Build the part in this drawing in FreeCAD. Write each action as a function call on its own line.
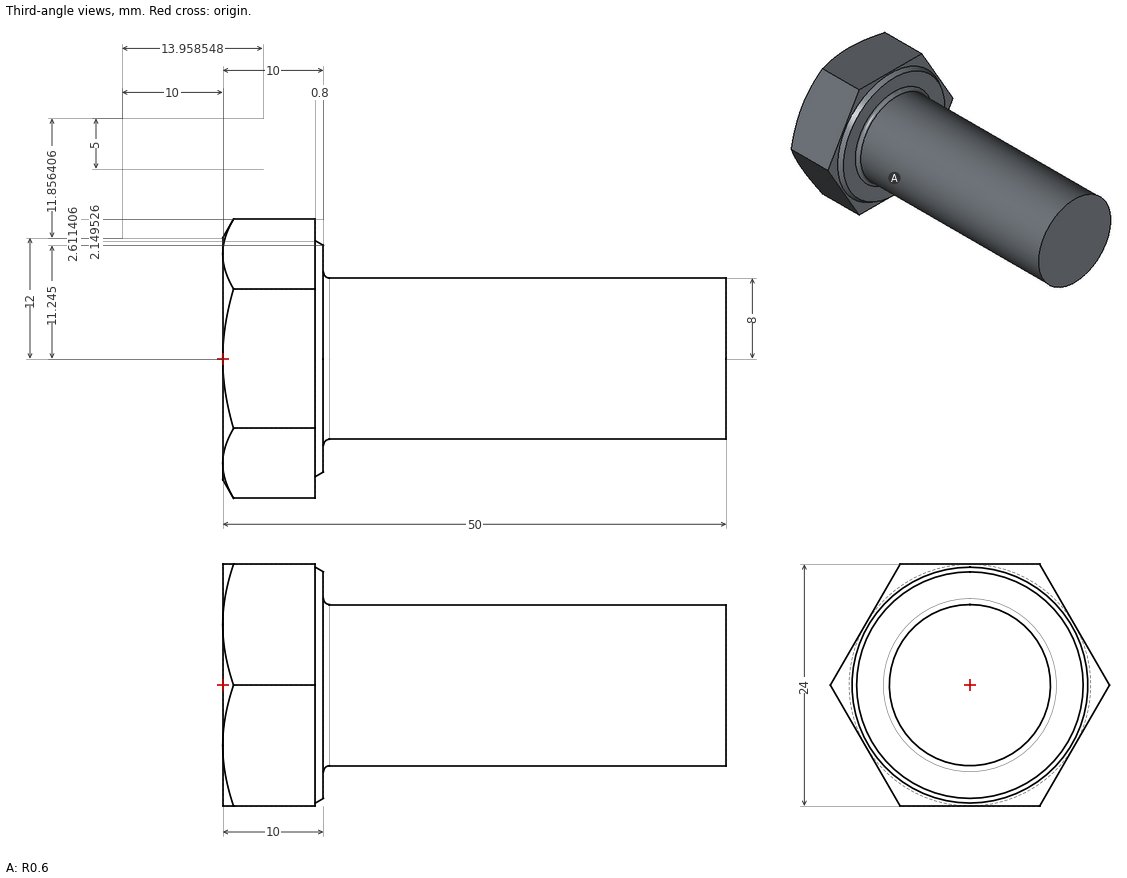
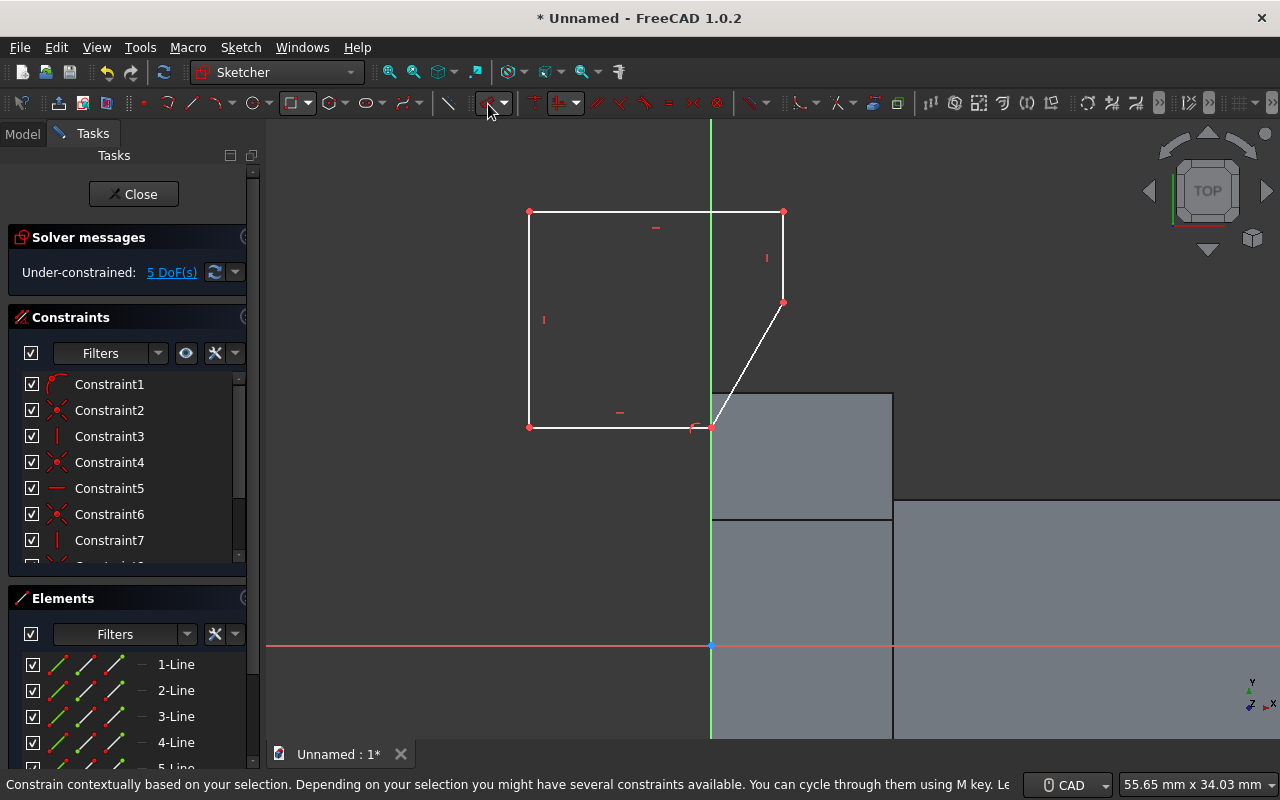
click(783, 276)
click(817, 257)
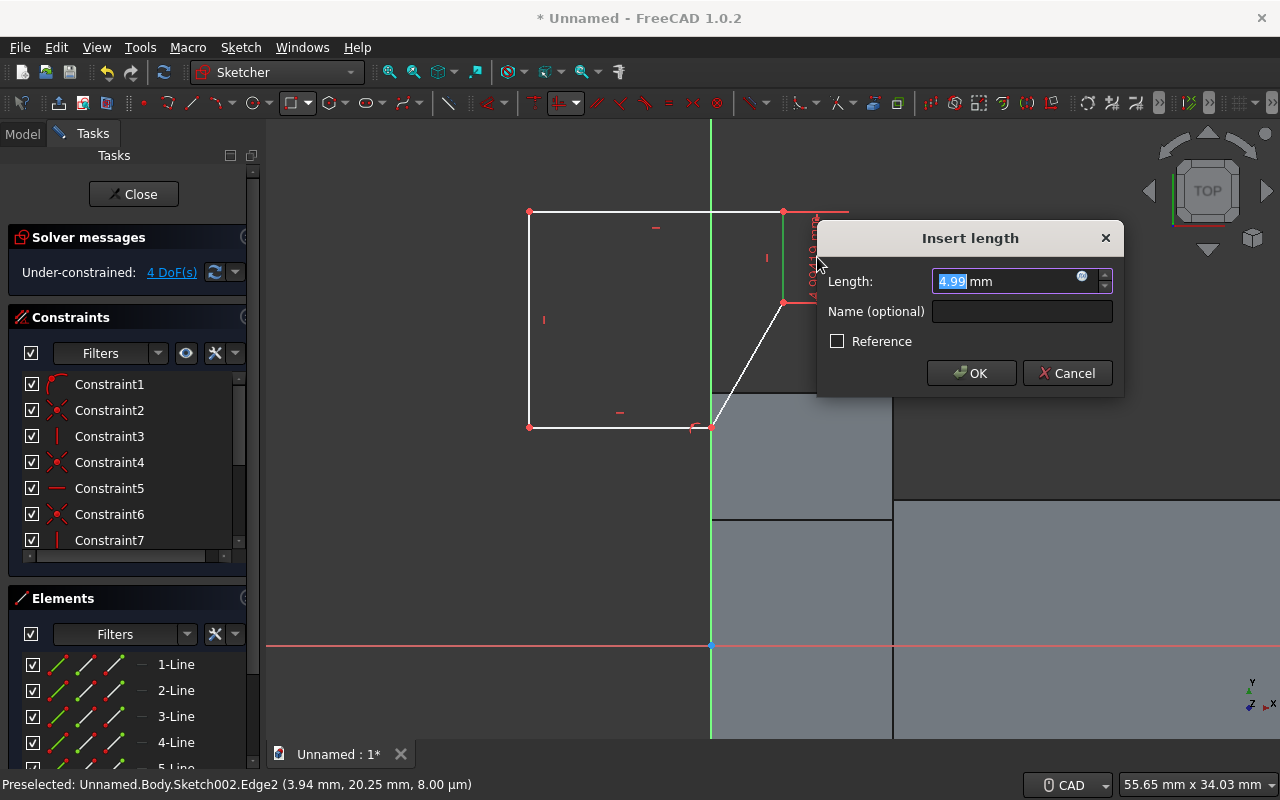
text(5)
key(Return)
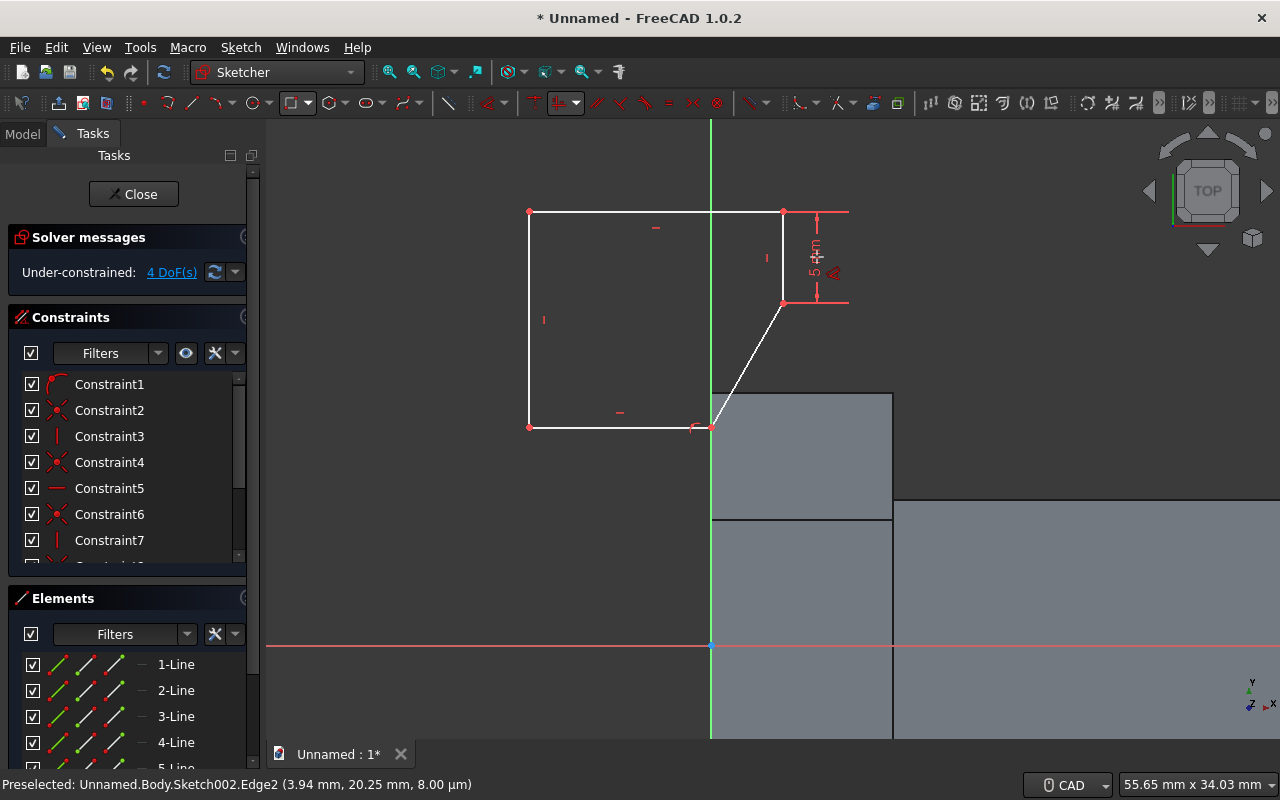
click(584, 428)
click(620, 394)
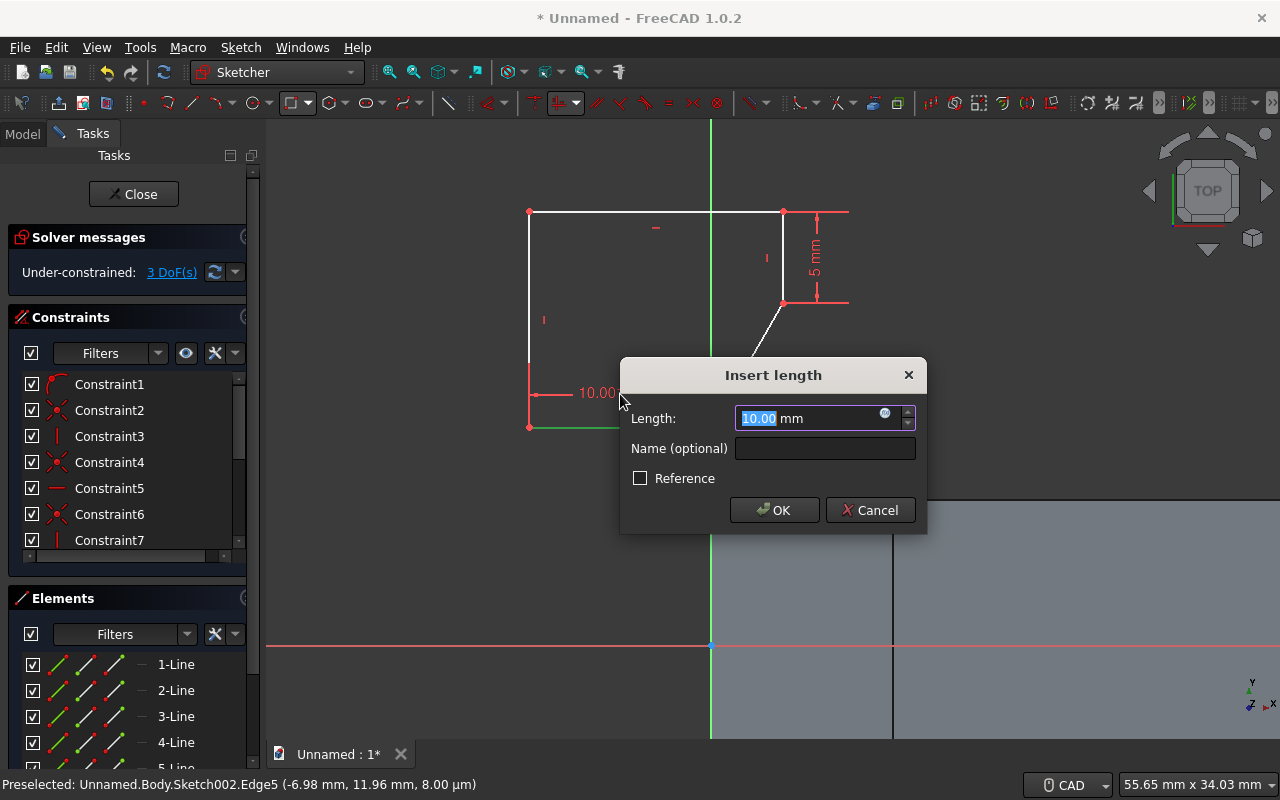
text(10)
key(Return)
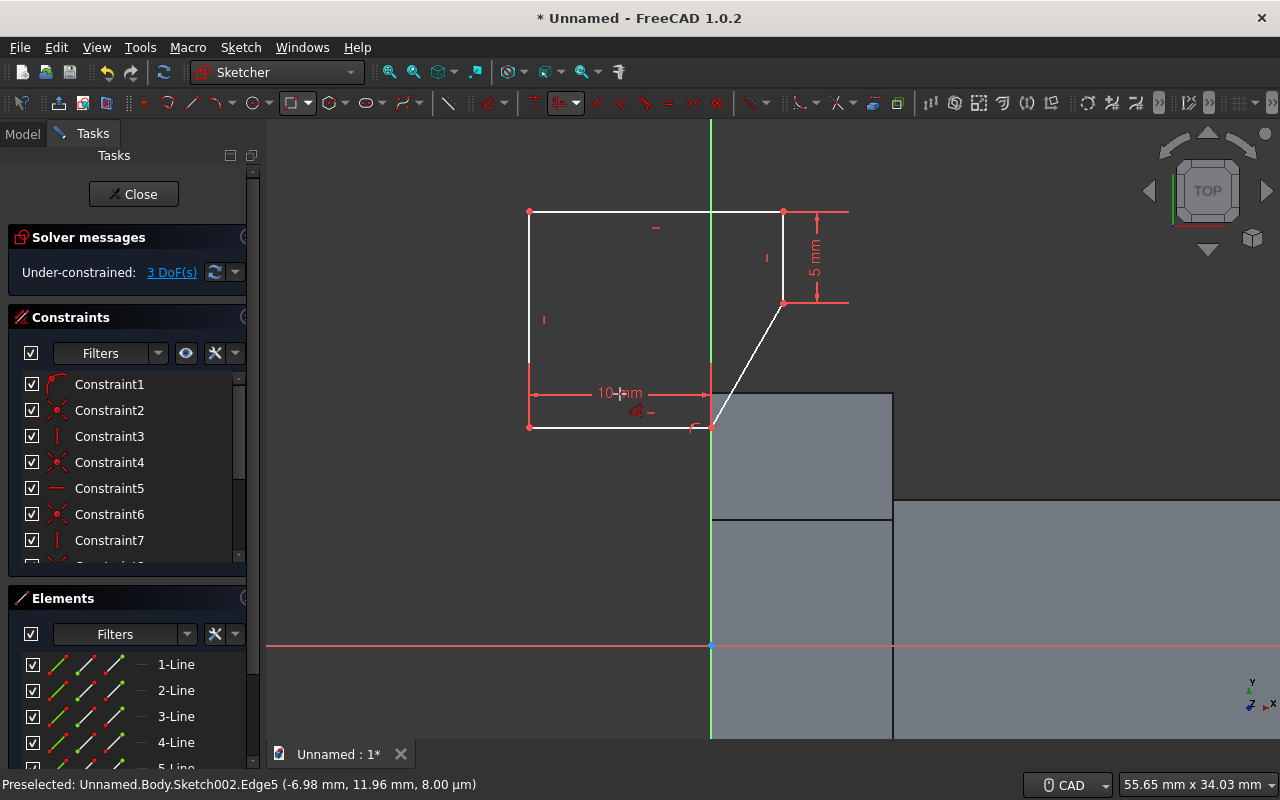
click(711, 428)
click(745, 537)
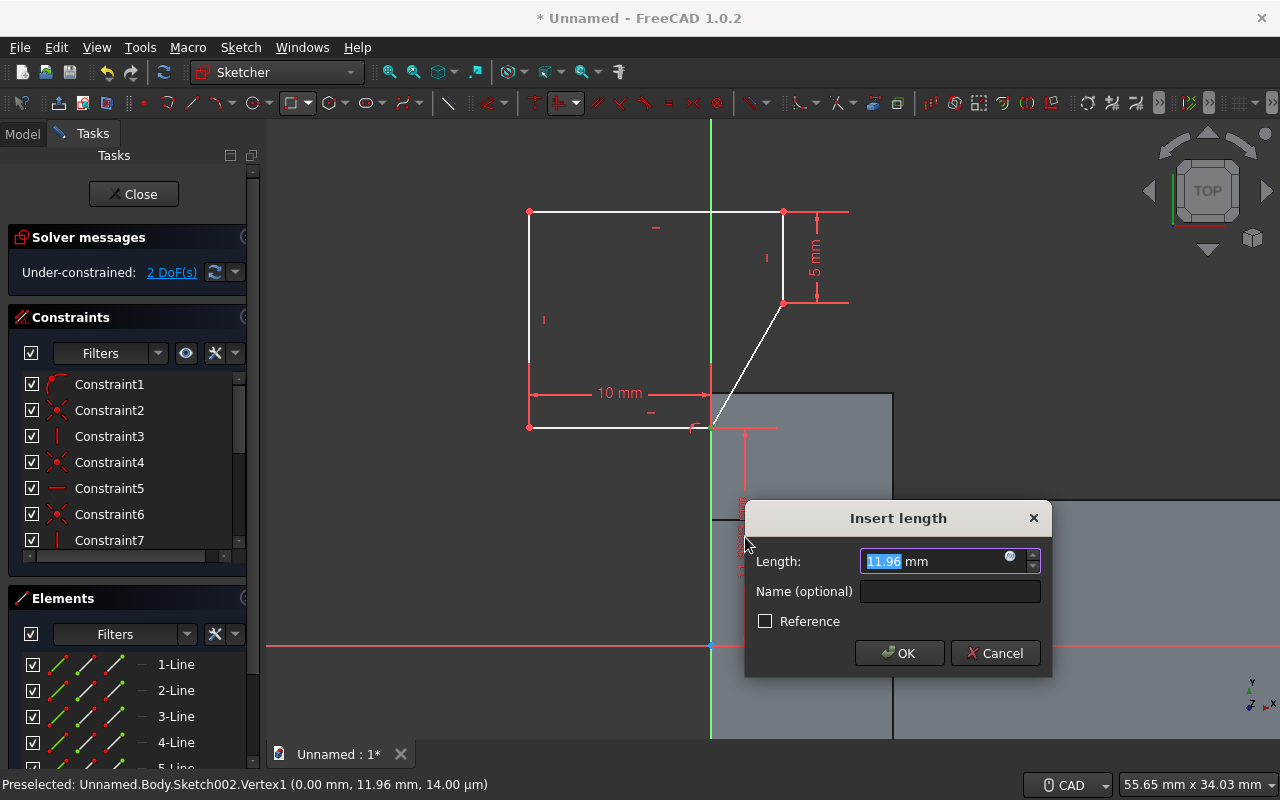
text(12)
key(Return)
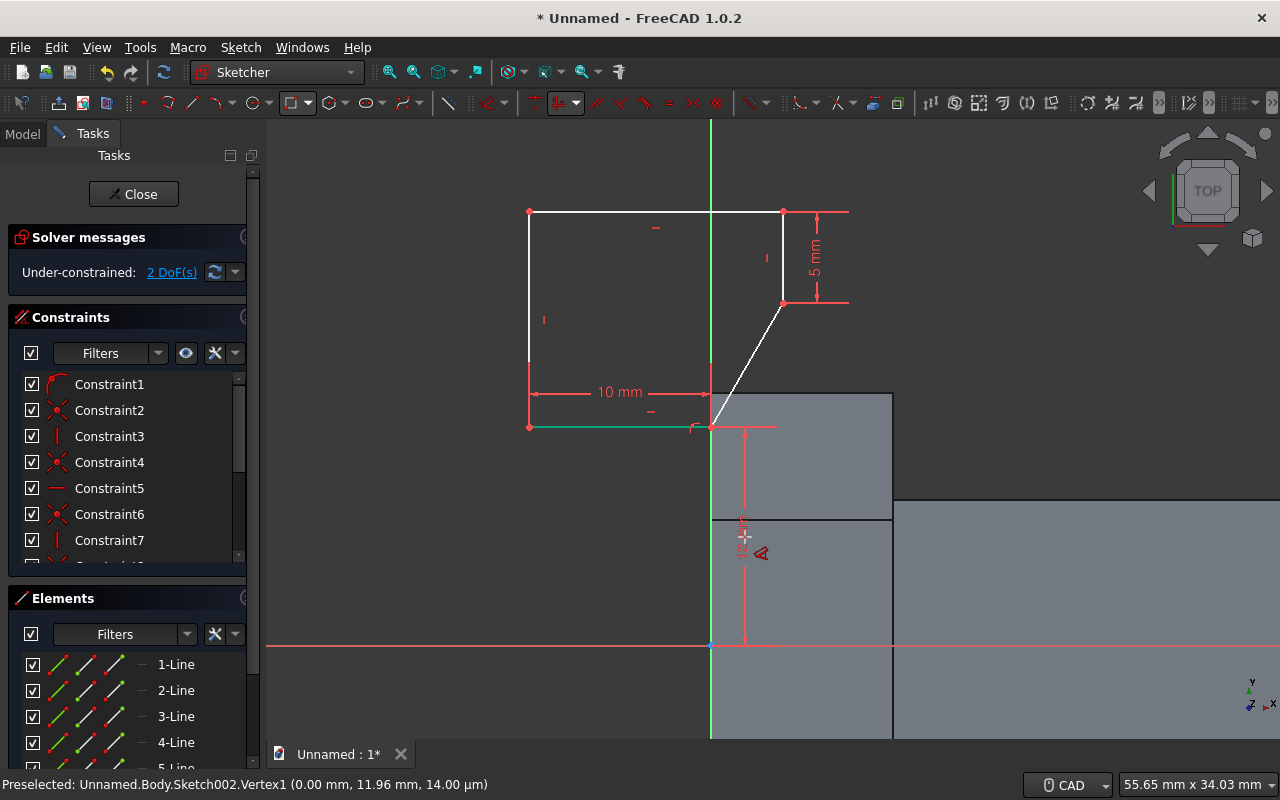
click(605, 212)
click(656, 178)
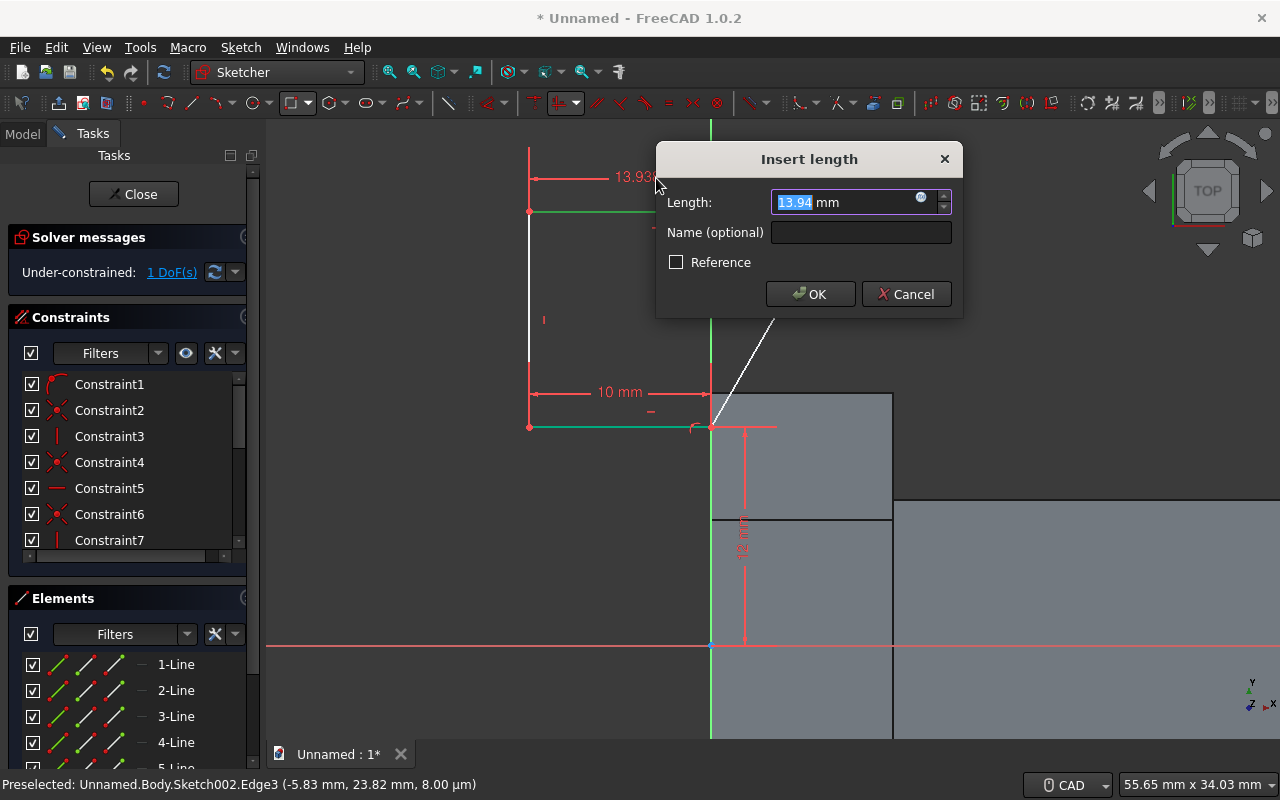
text(13.958548)
key(Return)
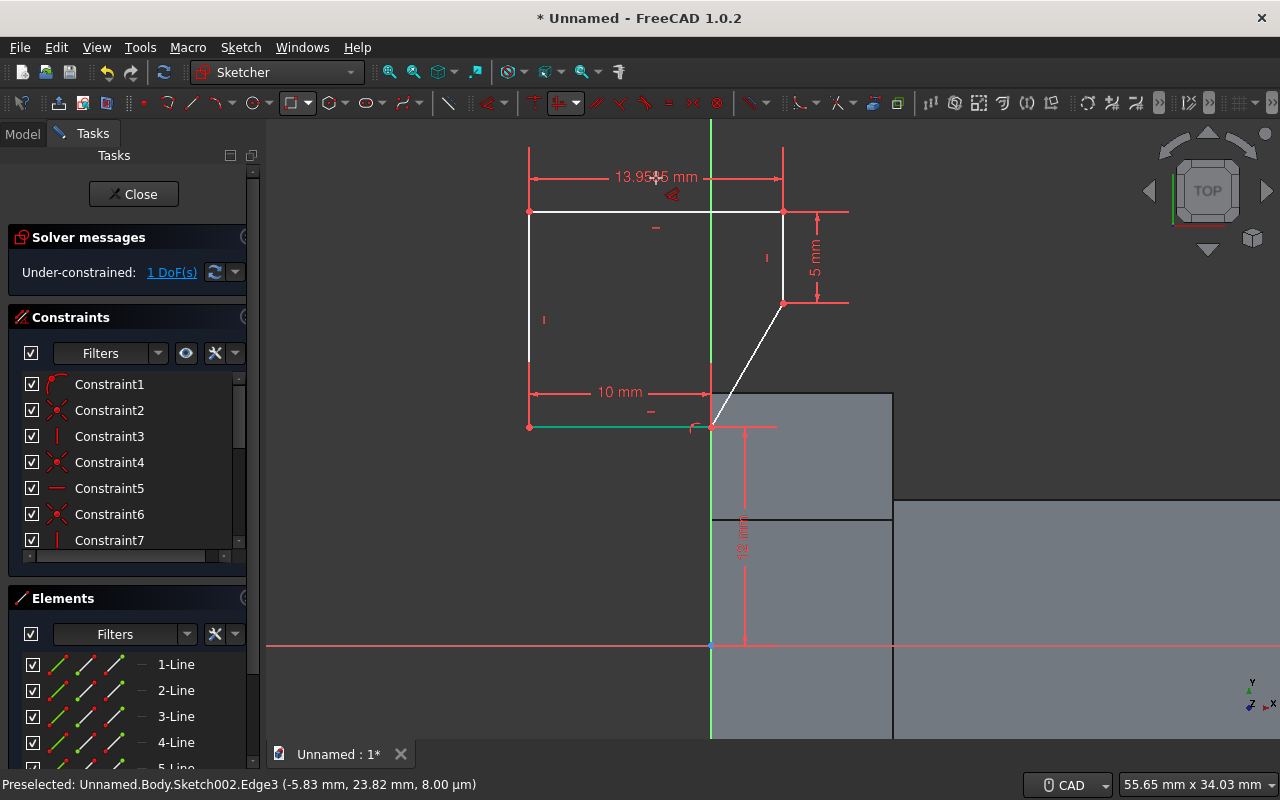
click(529, 277)
click(495, 320)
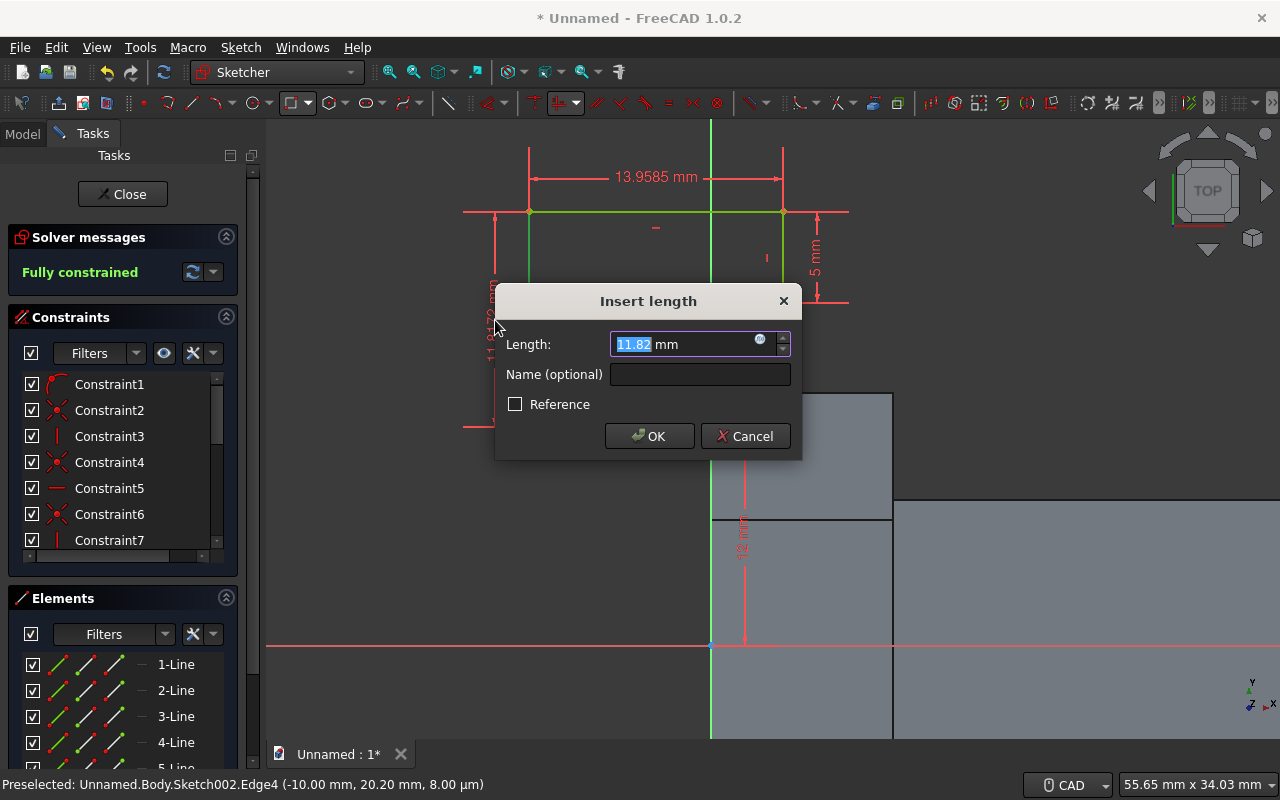
text(11.856406)
key(Return)
key(Escape)